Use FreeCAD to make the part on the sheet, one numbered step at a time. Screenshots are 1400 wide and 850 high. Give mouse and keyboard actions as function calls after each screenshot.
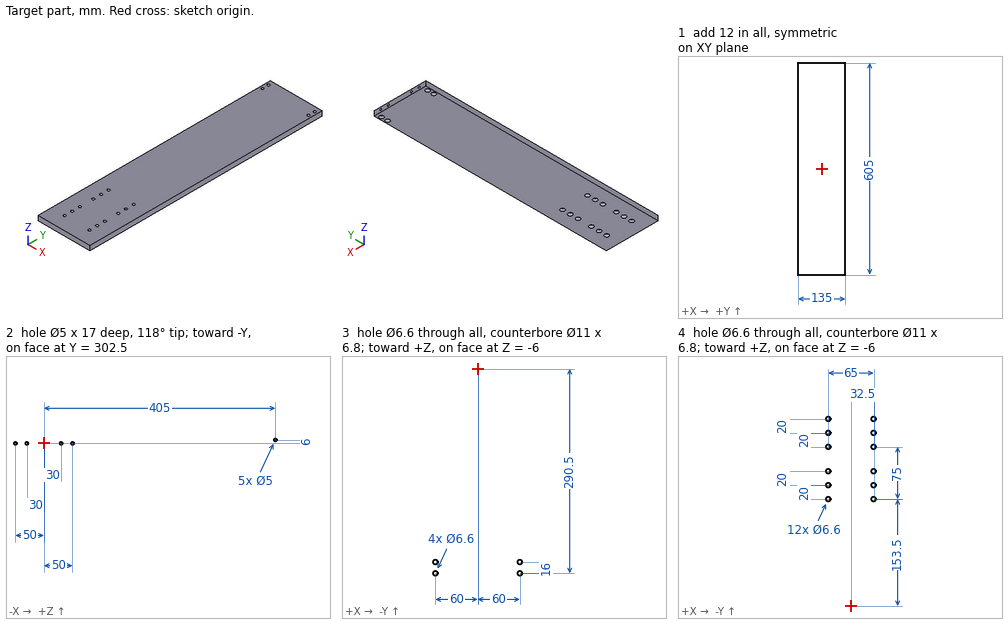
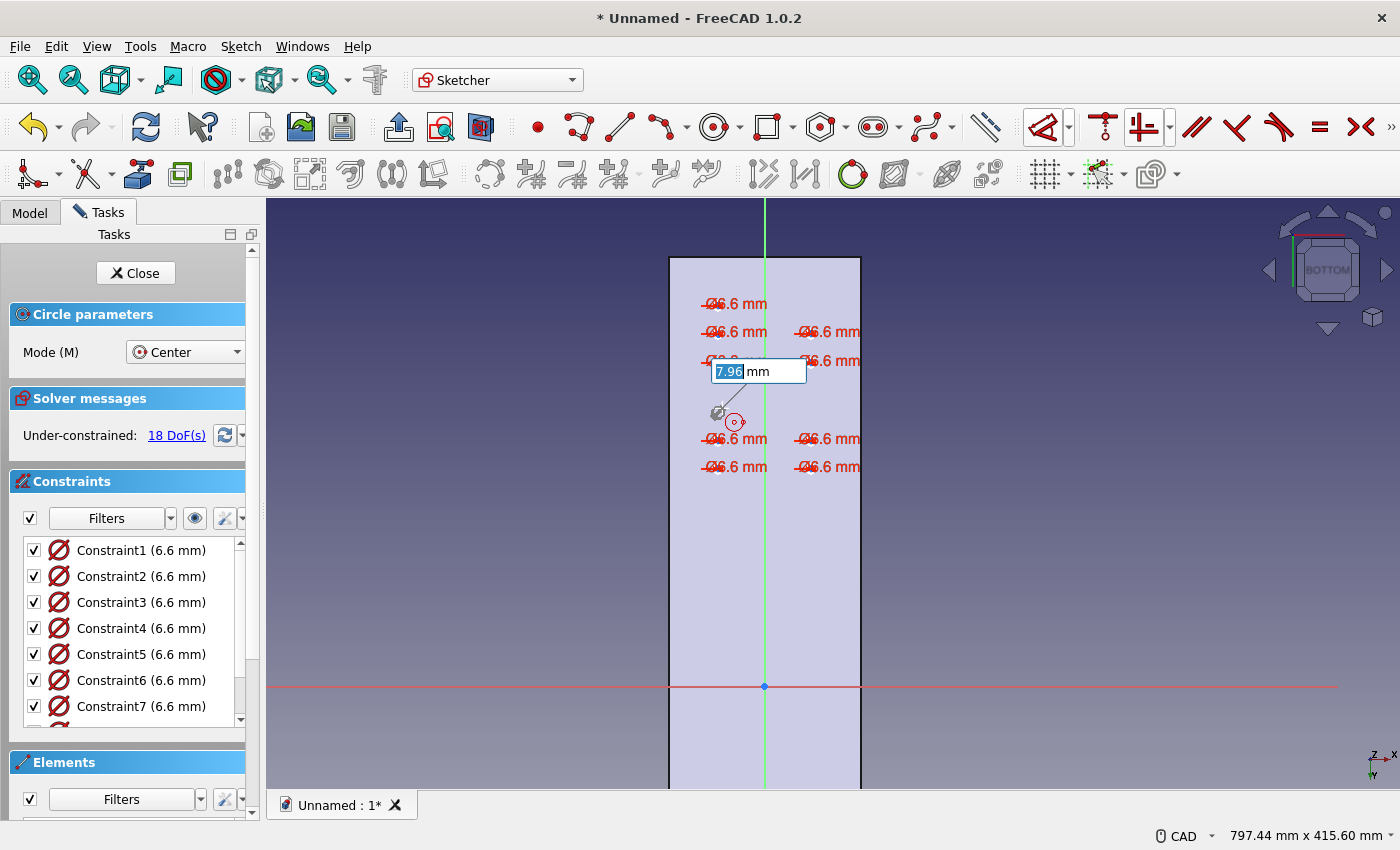
text(6.6)
key(Return)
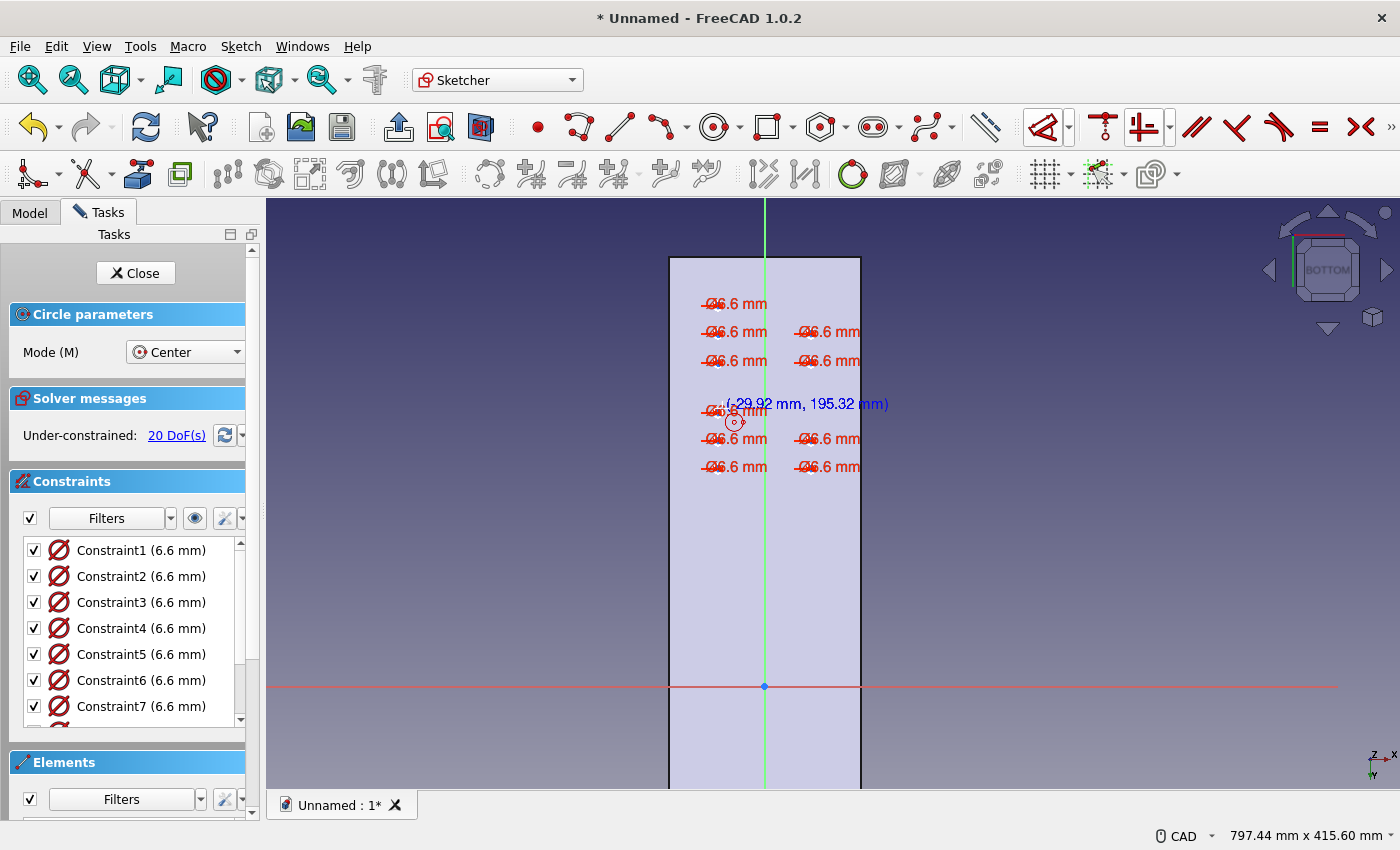
scroll(811, 412, up, 8)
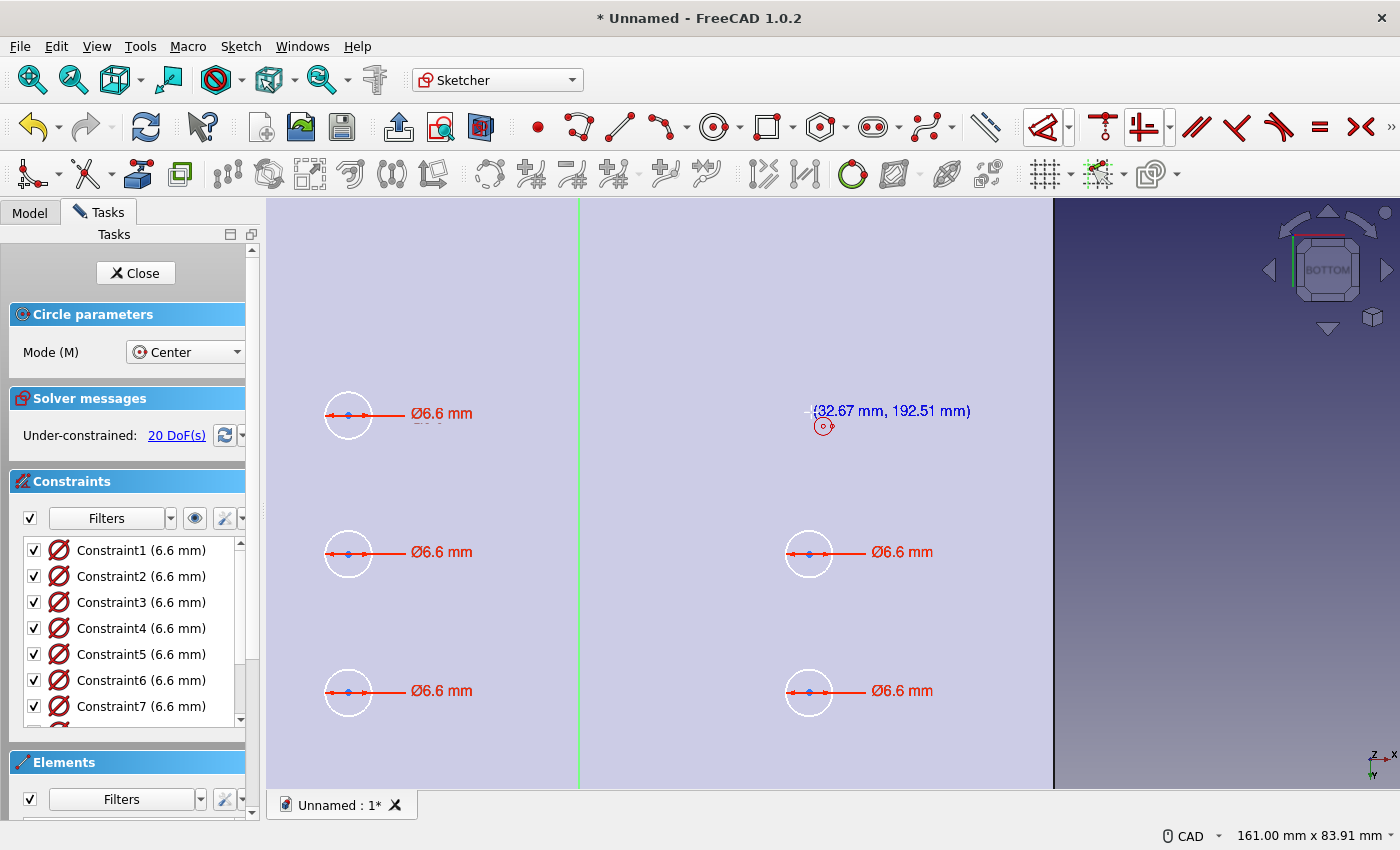
scroll(811, 412, down, 8)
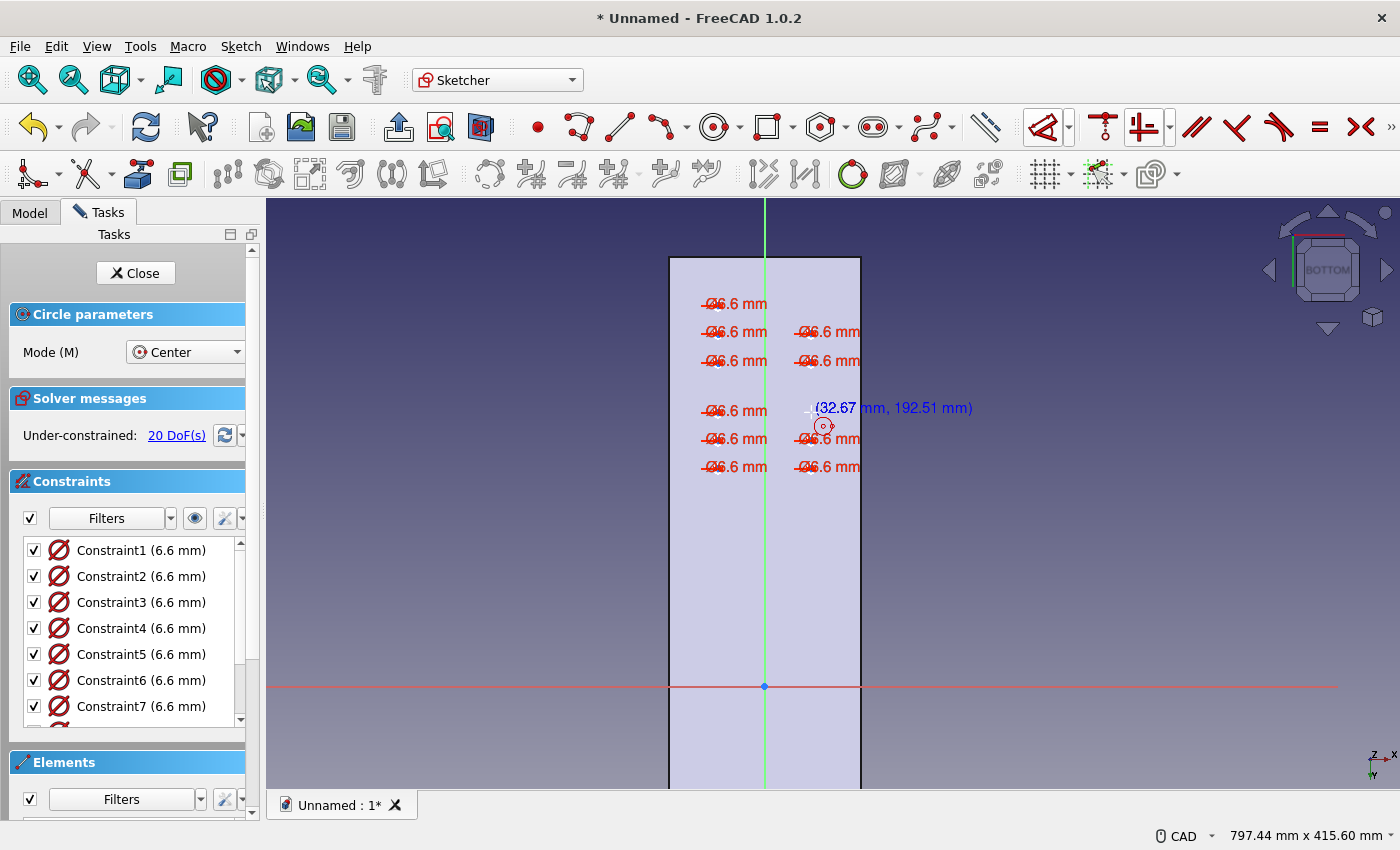
click(811, 412)
move(814, 408)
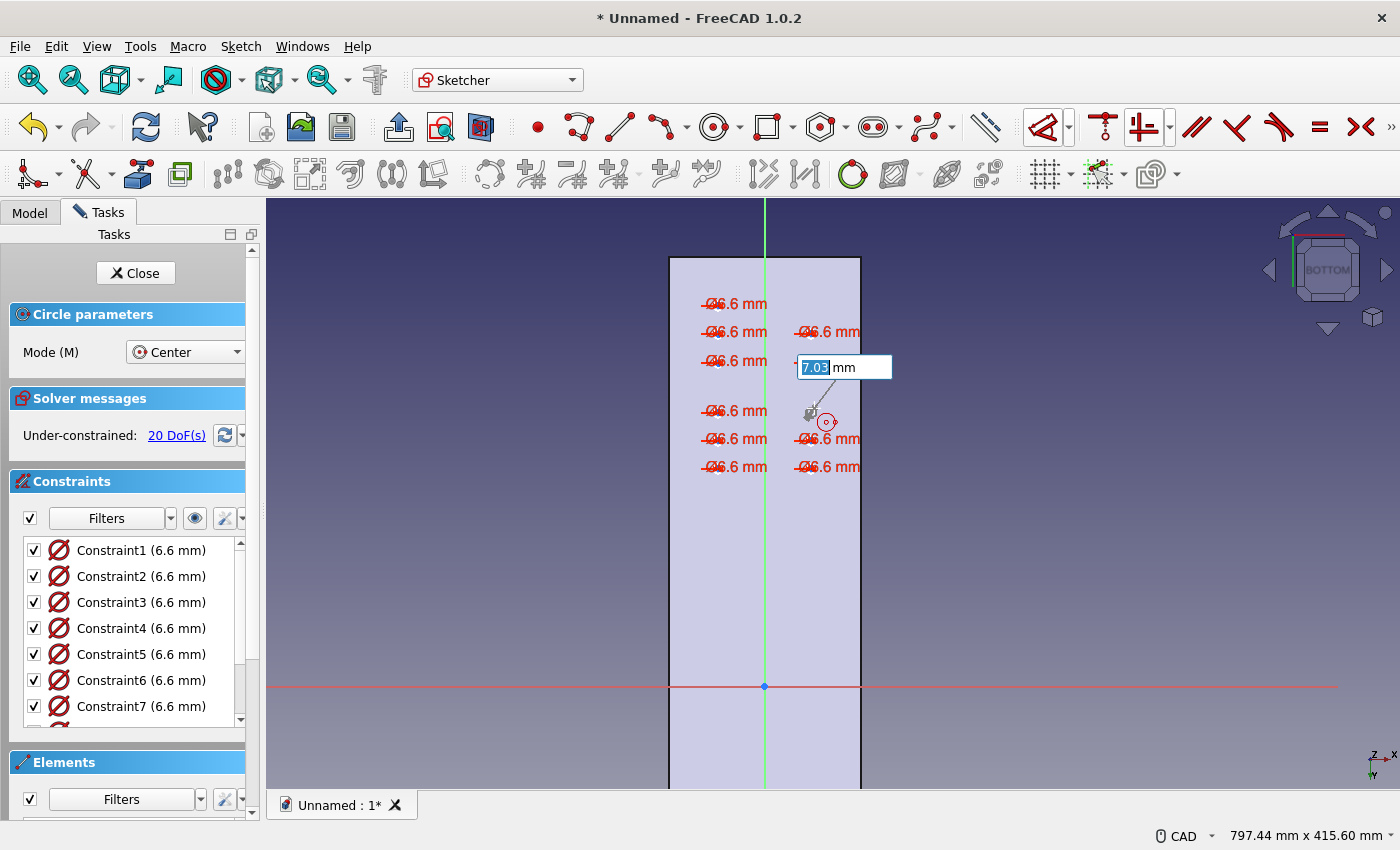
text(6.6)
key(Return)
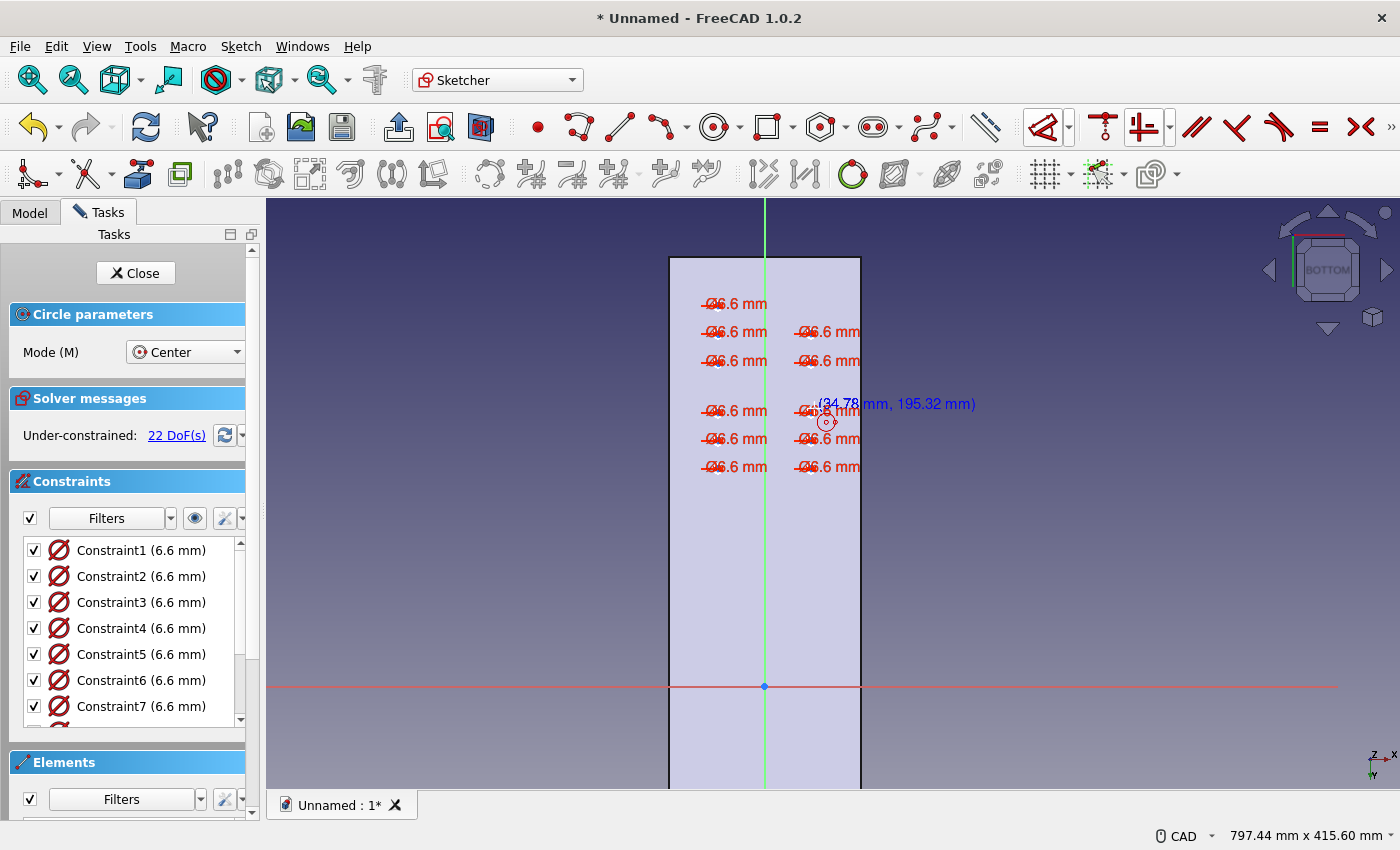
scroll(811, 305, up, 8)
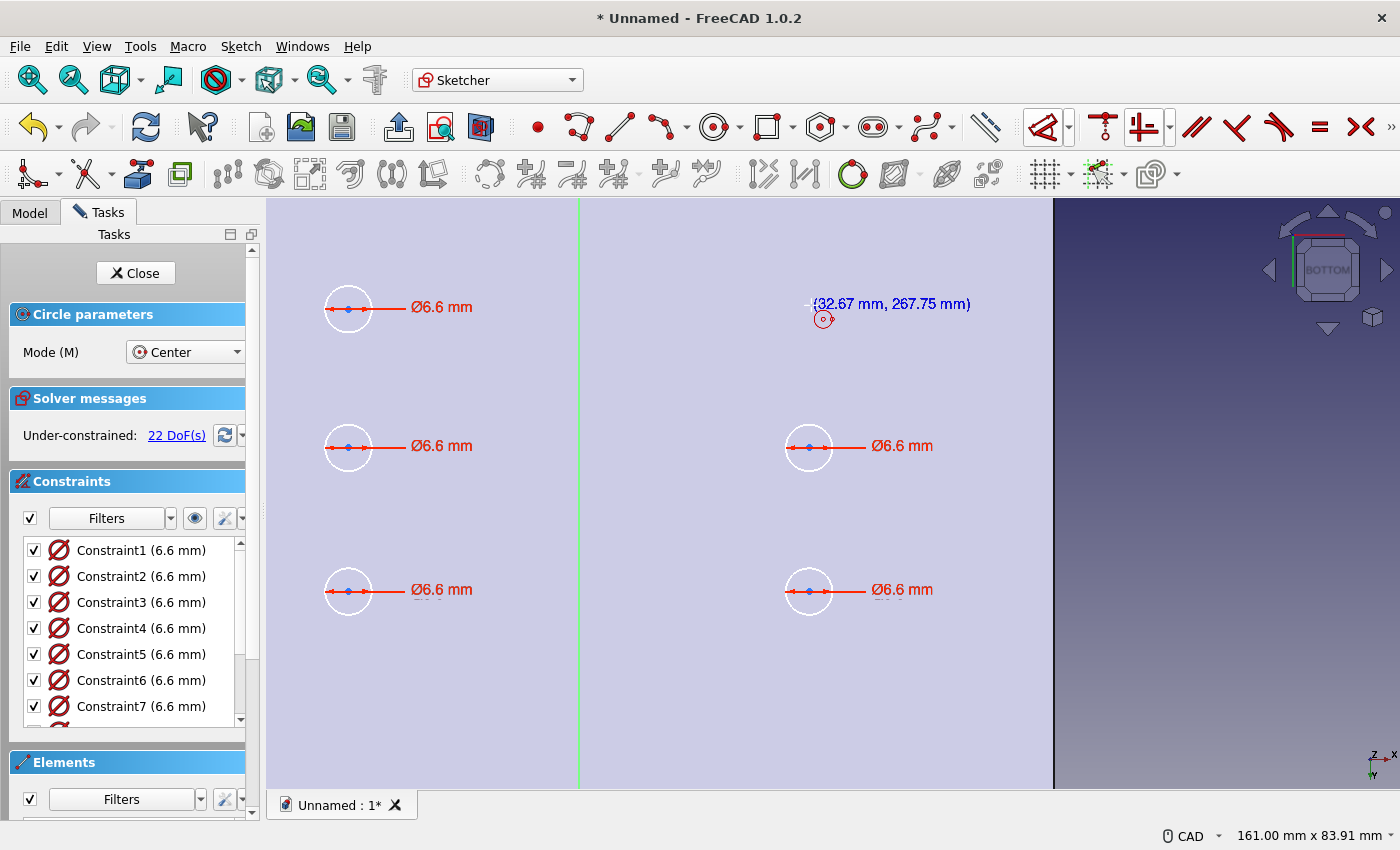
scroll(811, 305, down, 8)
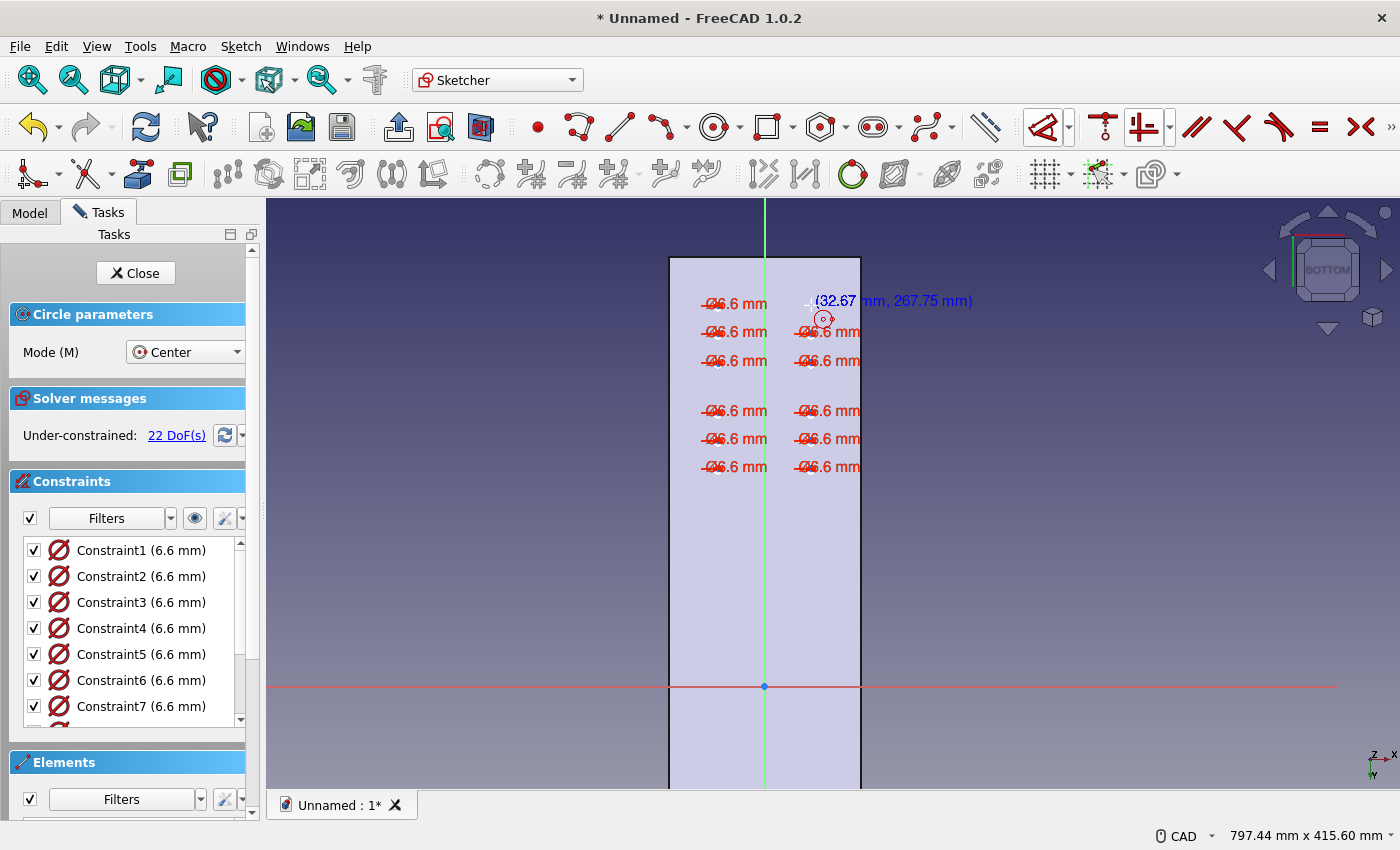
click(811, 305)
move(814, 302)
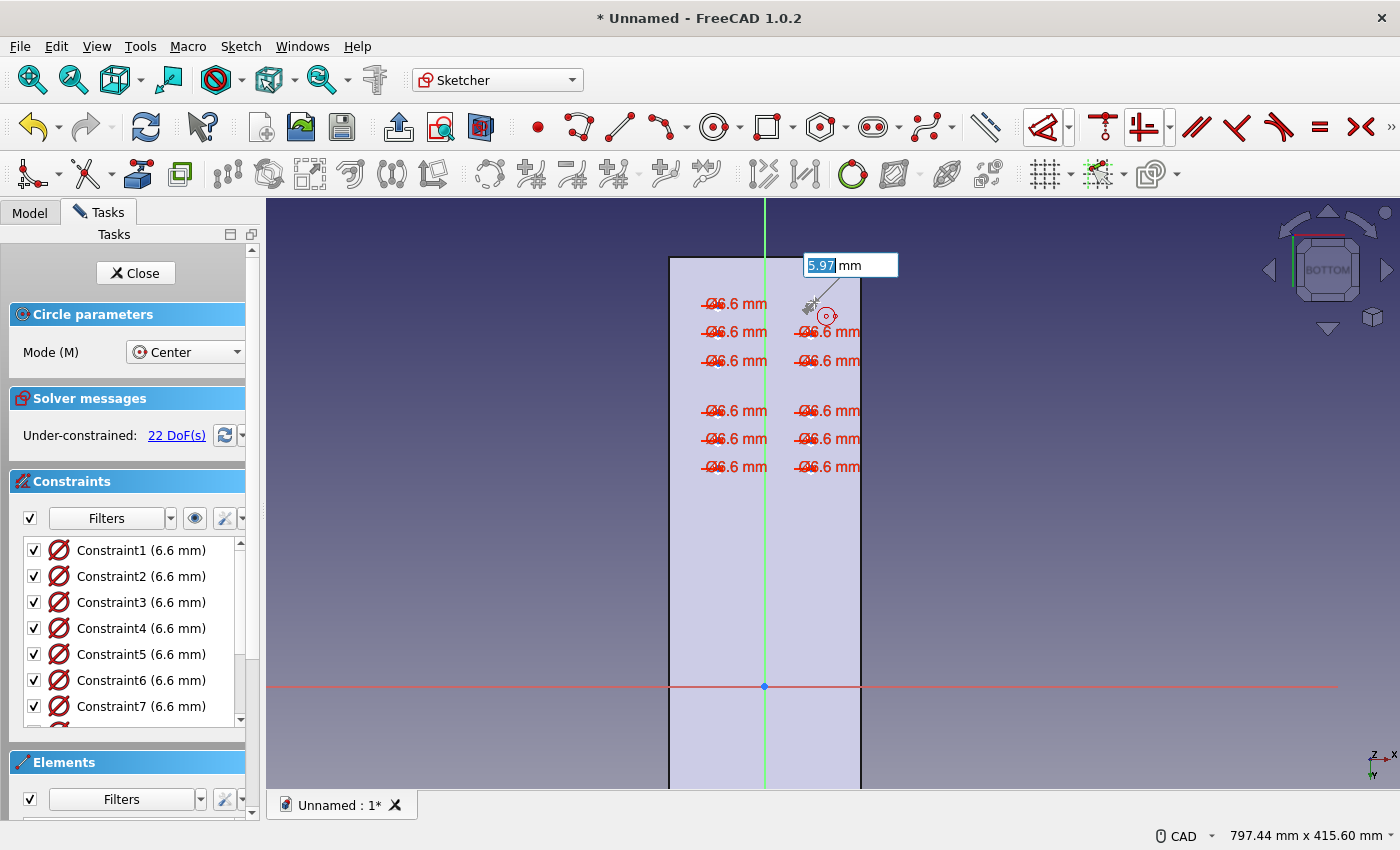
text(6.6)
key(Return)
key(Escape)